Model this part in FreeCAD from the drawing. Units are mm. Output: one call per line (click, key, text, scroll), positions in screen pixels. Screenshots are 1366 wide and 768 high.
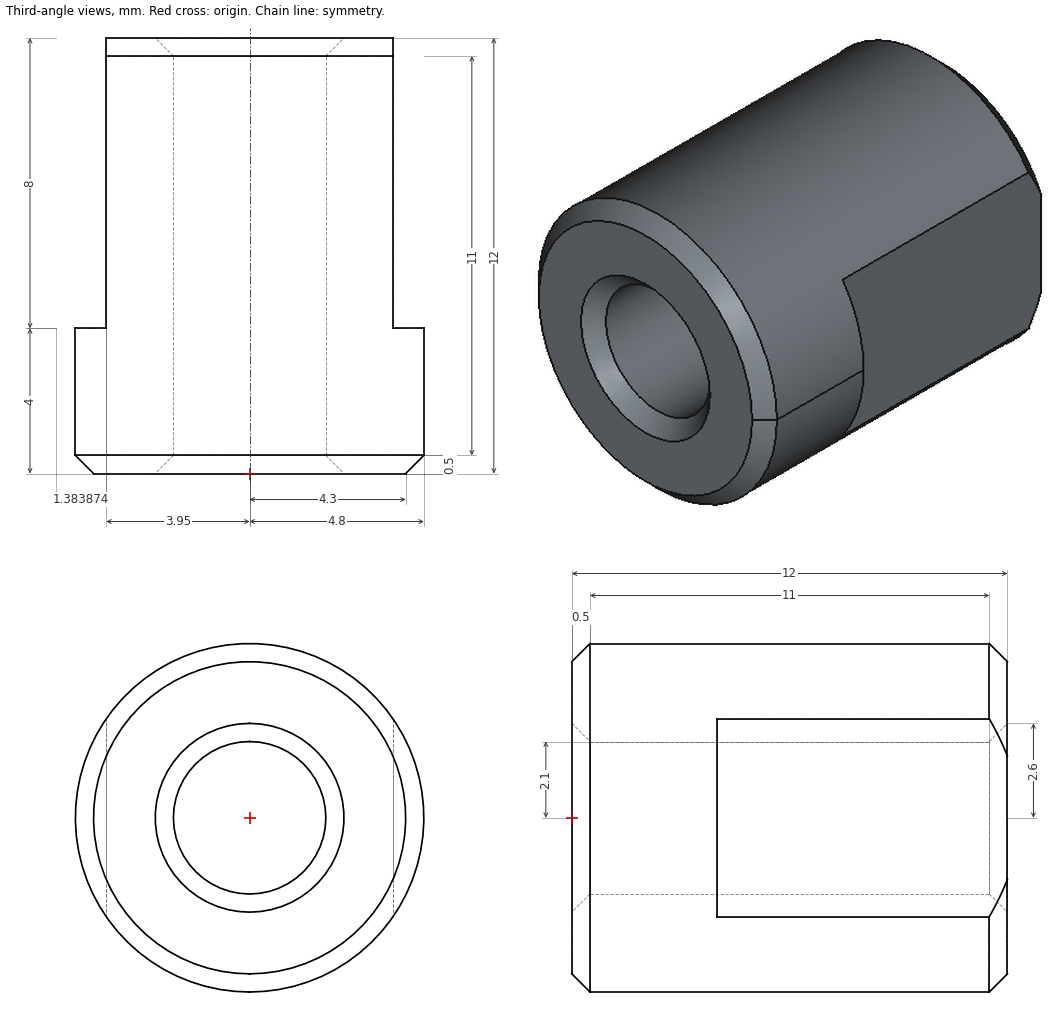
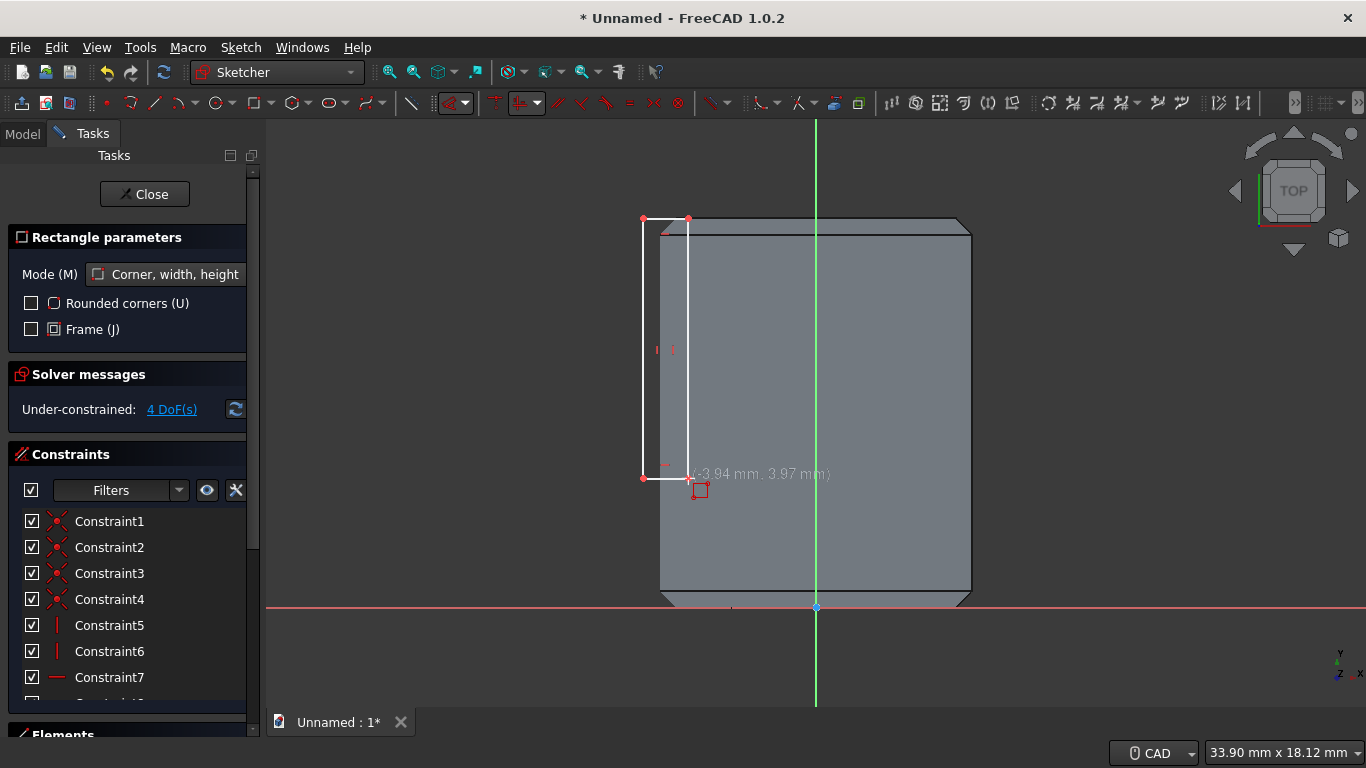
click(944, 218)
click(989, 478)
key(Escape)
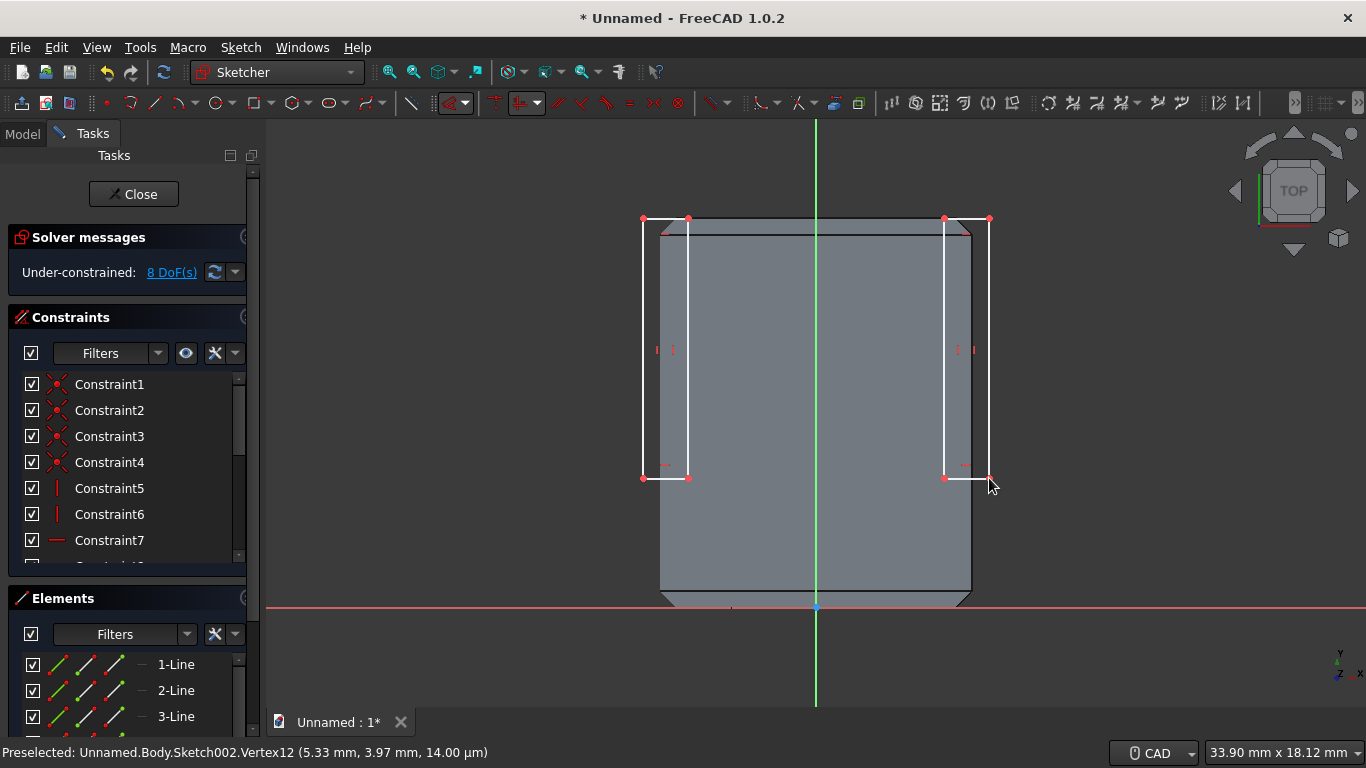
click(688, 219)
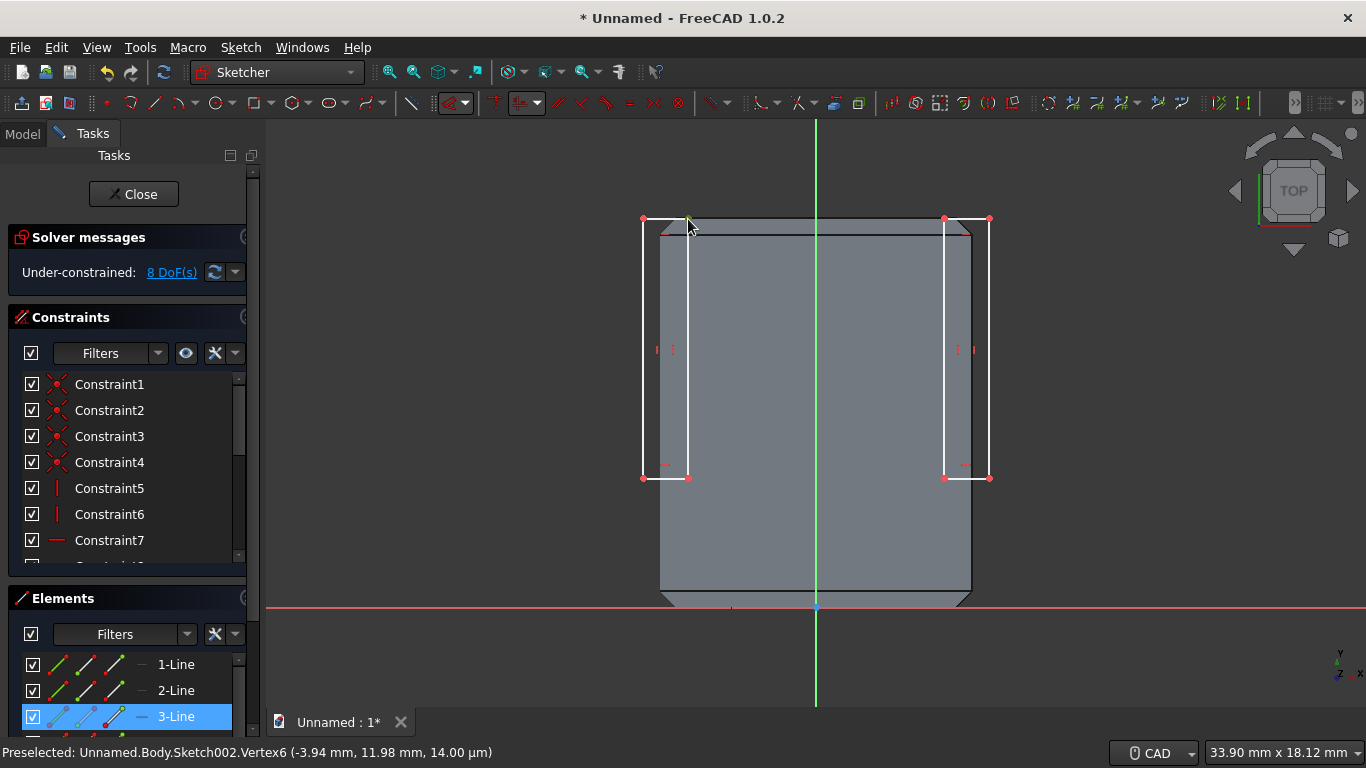
click(944, 219)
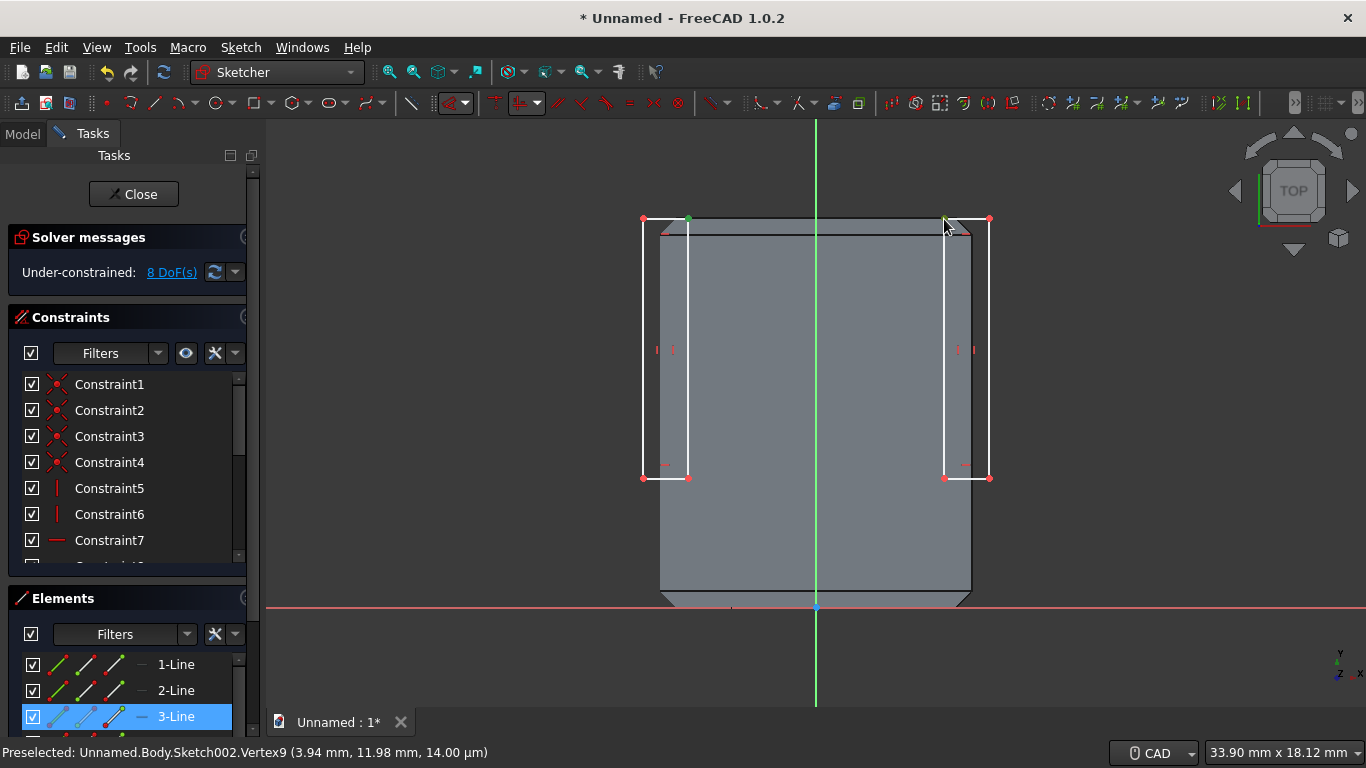
click(816, 641)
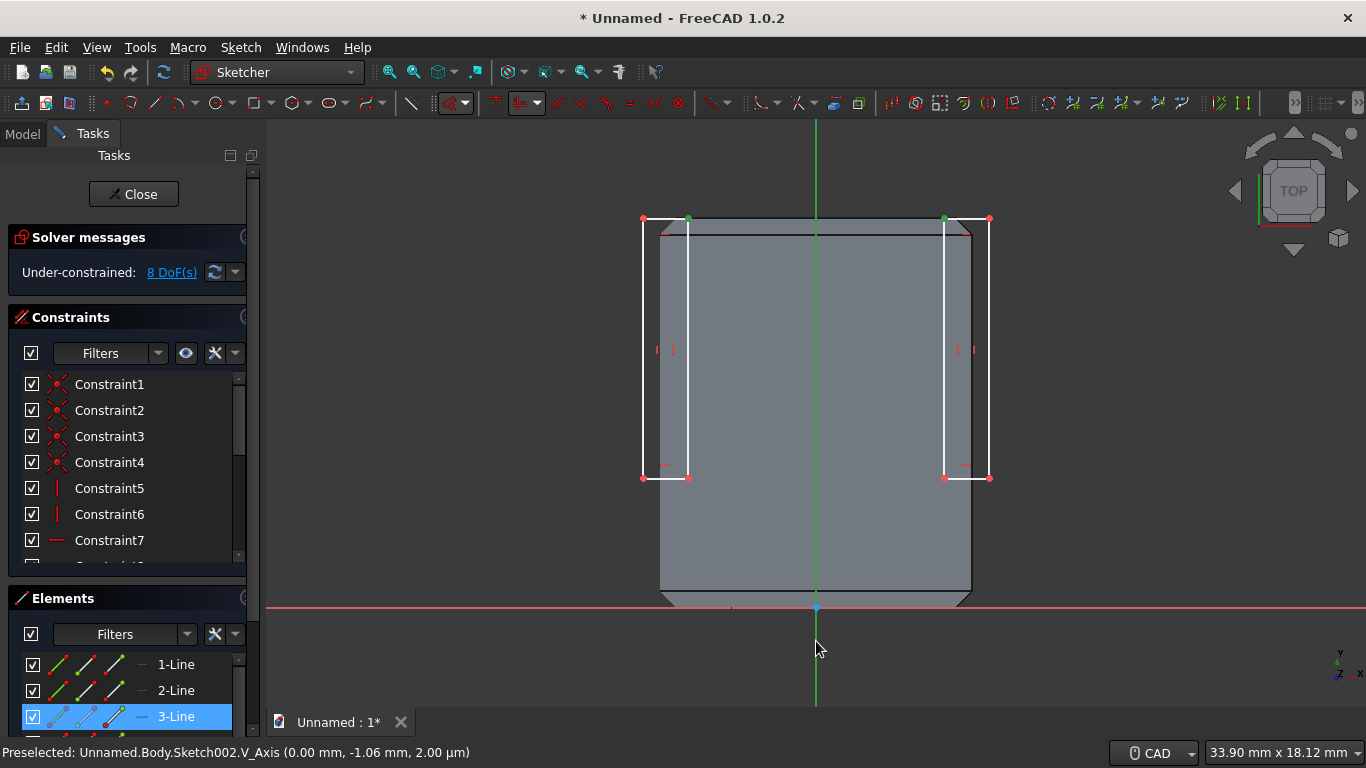
click(654, 104)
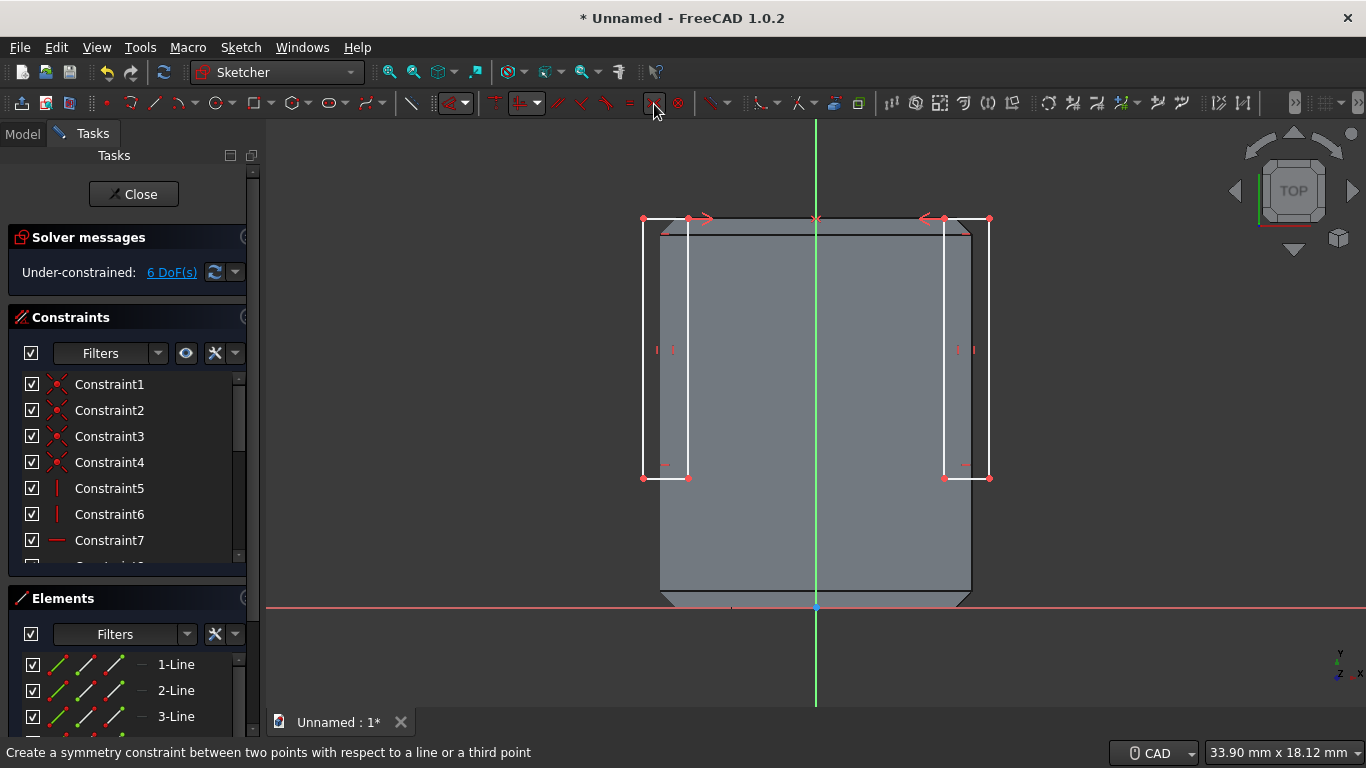
click(643, 479)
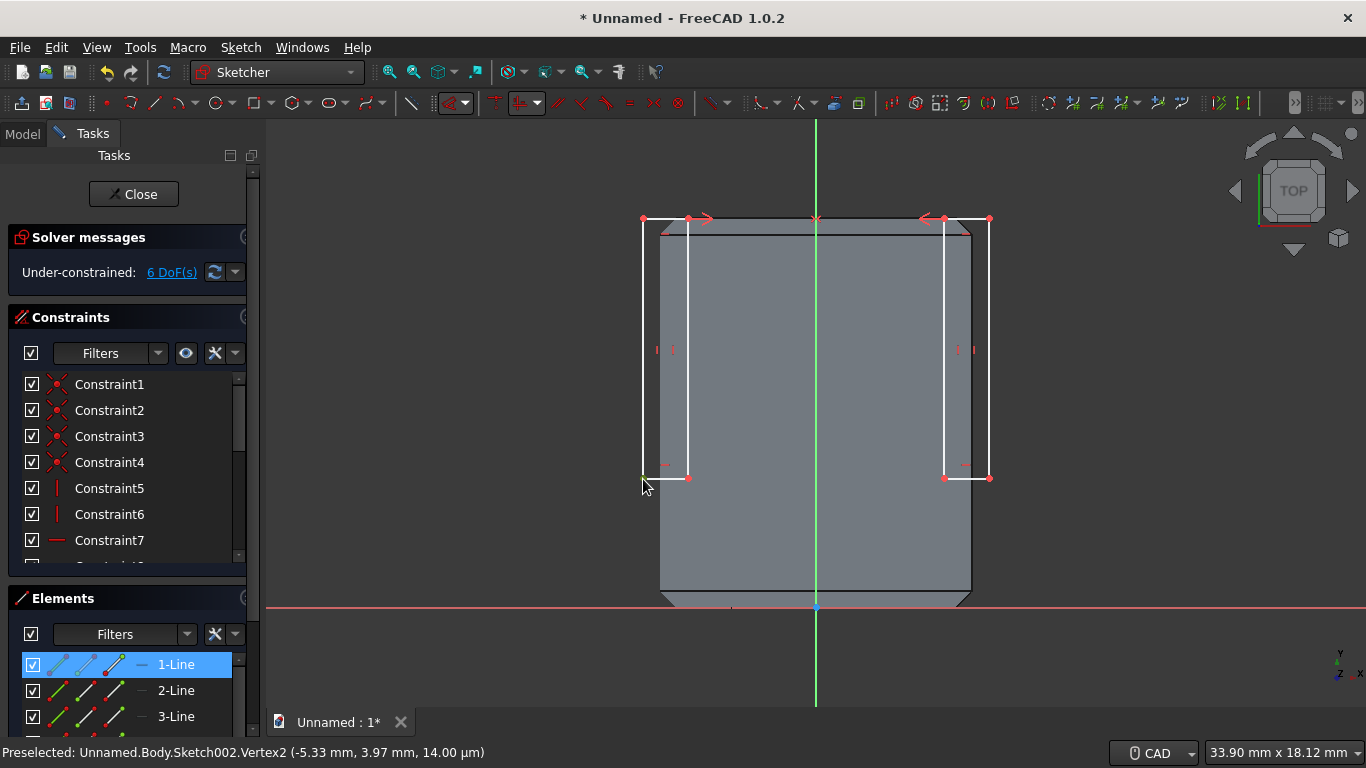
click(989, 479)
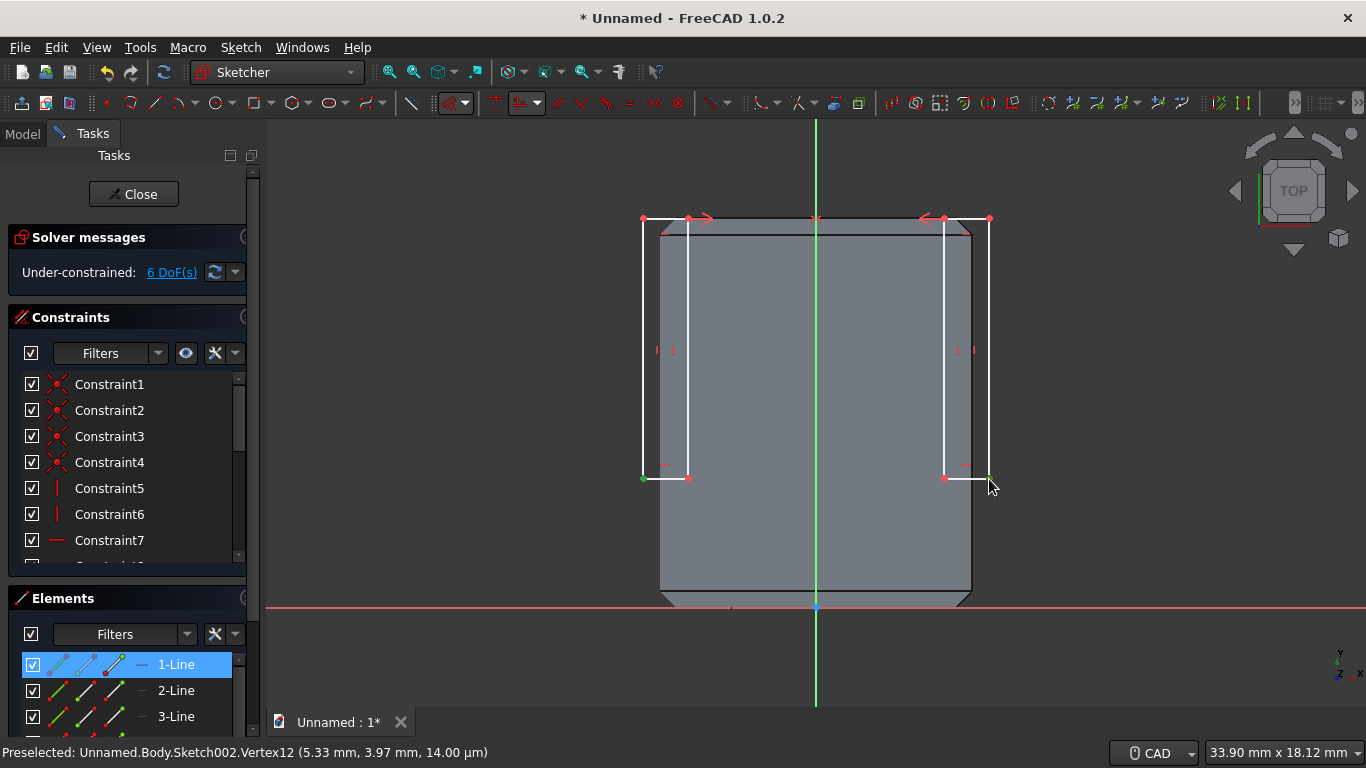
click(816, 641)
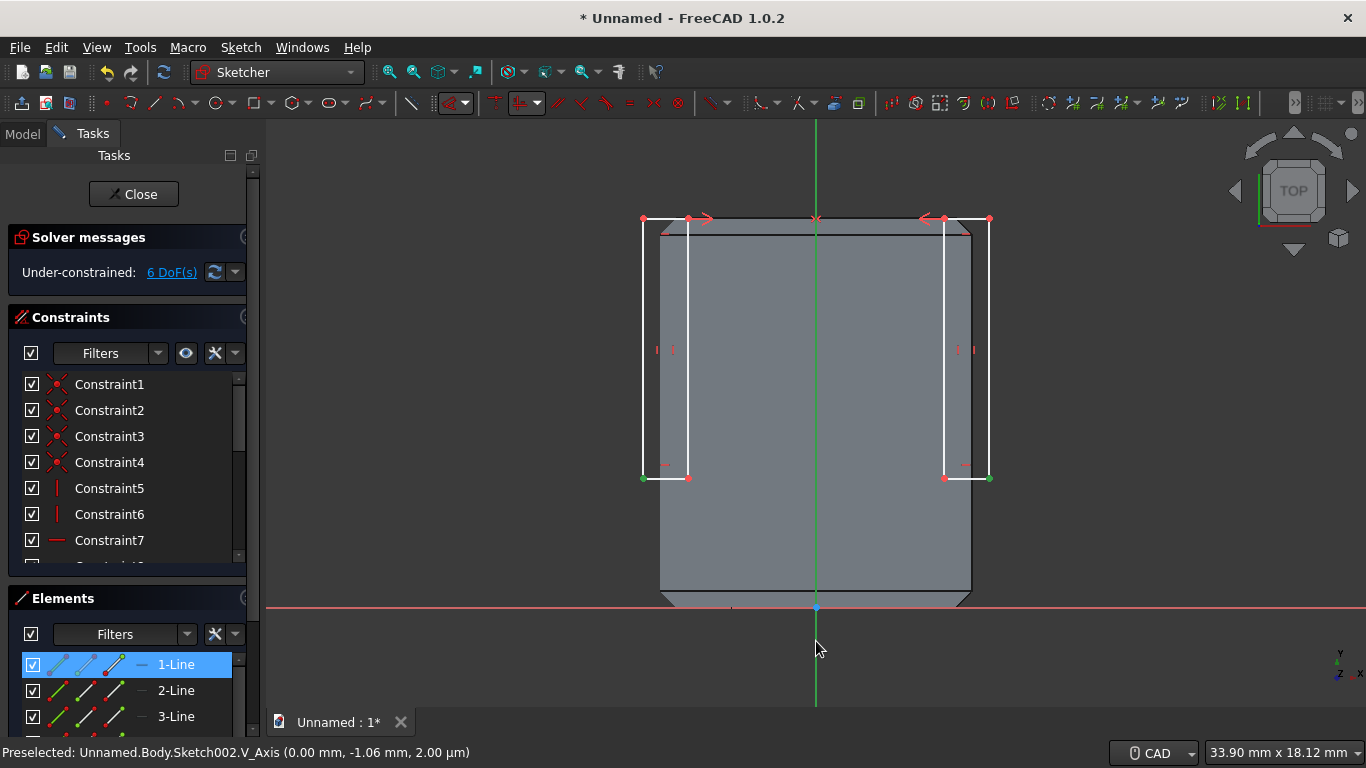
click(654, 104)